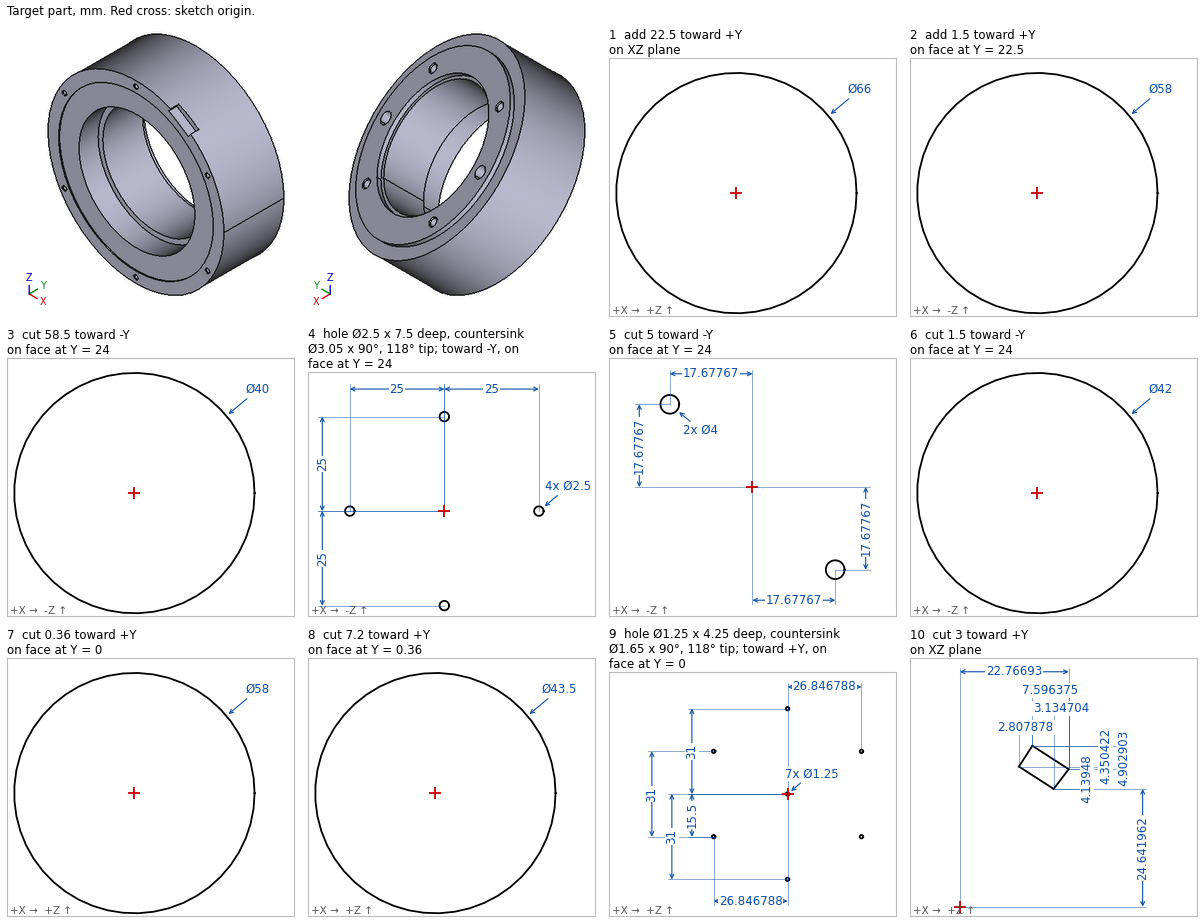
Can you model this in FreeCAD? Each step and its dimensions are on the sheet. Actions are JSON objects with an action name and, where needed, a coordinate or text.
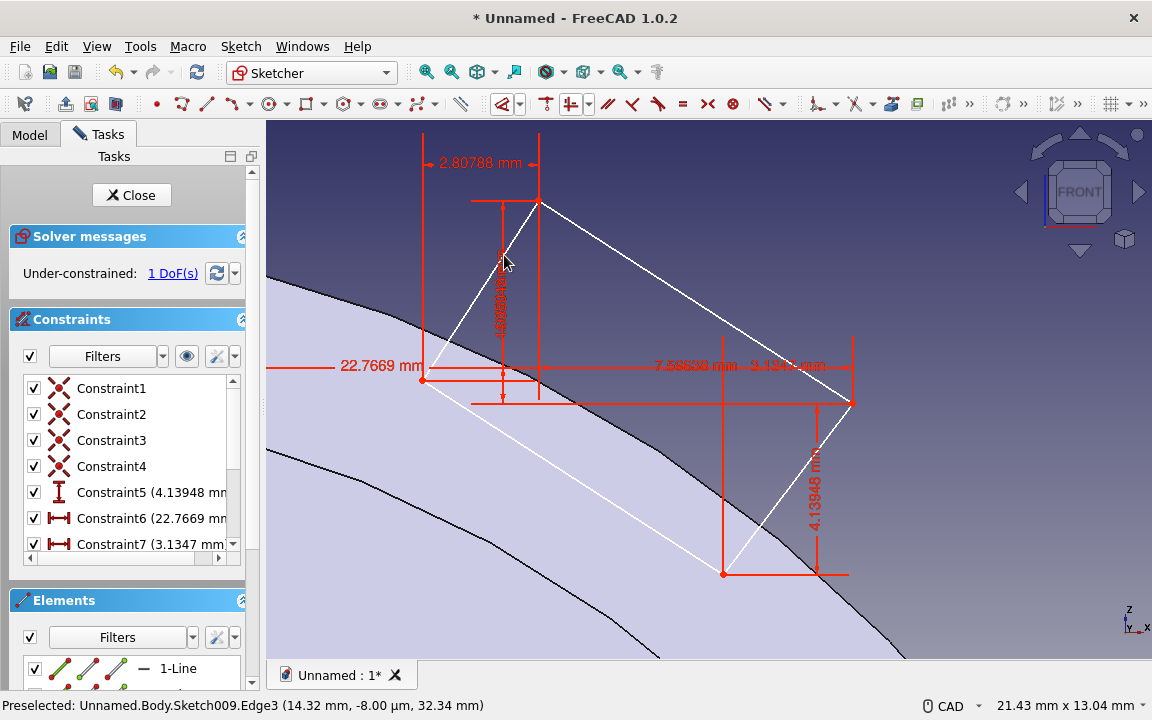
{"action": "left_click", "coordinate": [723, 575]}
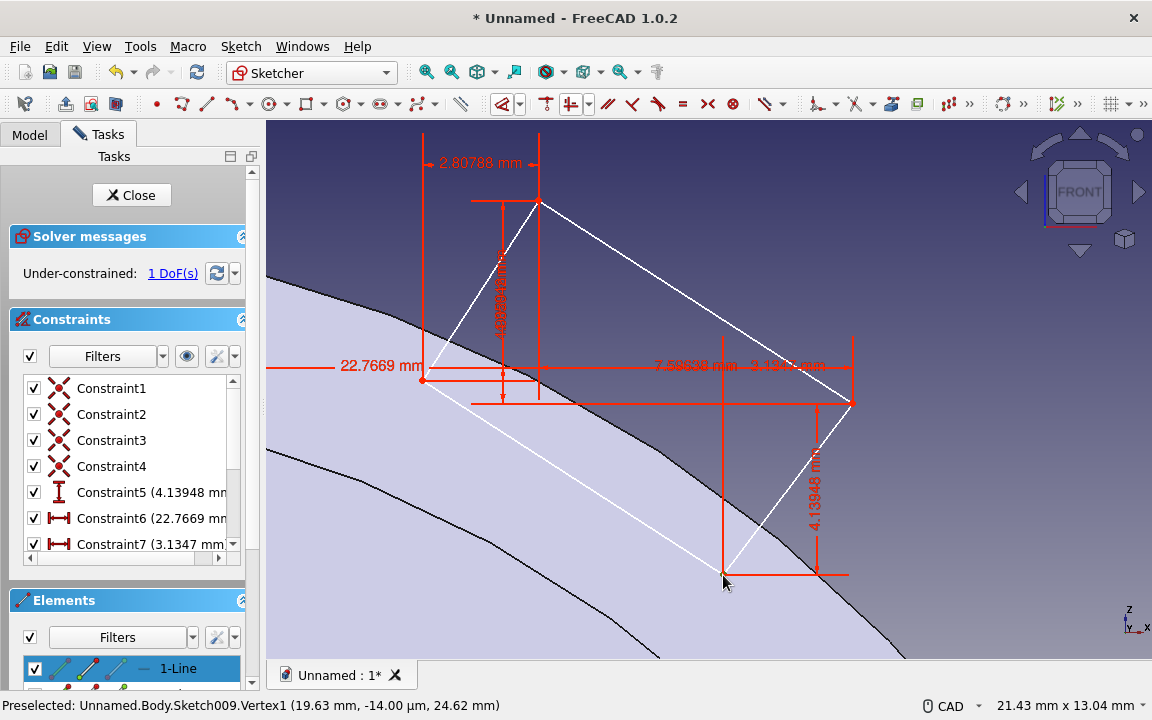
{"action": "key", "text": "i"}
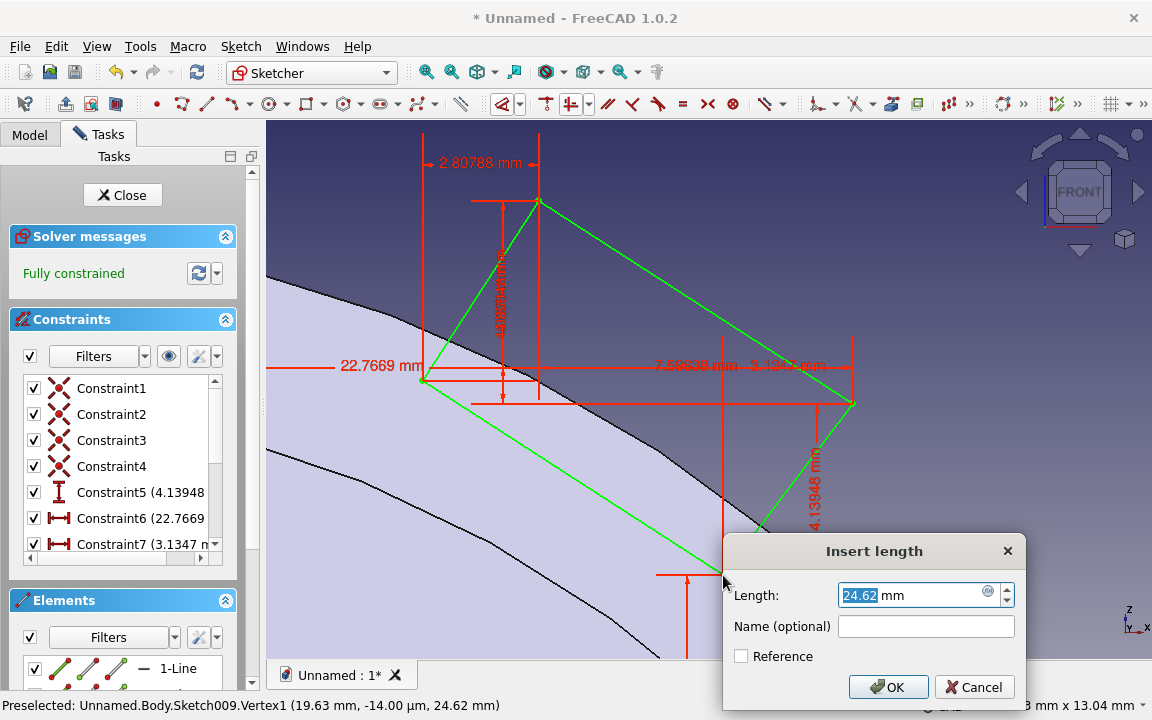
{"action": "type", "text": "24.641962"}
{"action": "key", "text": "Return"}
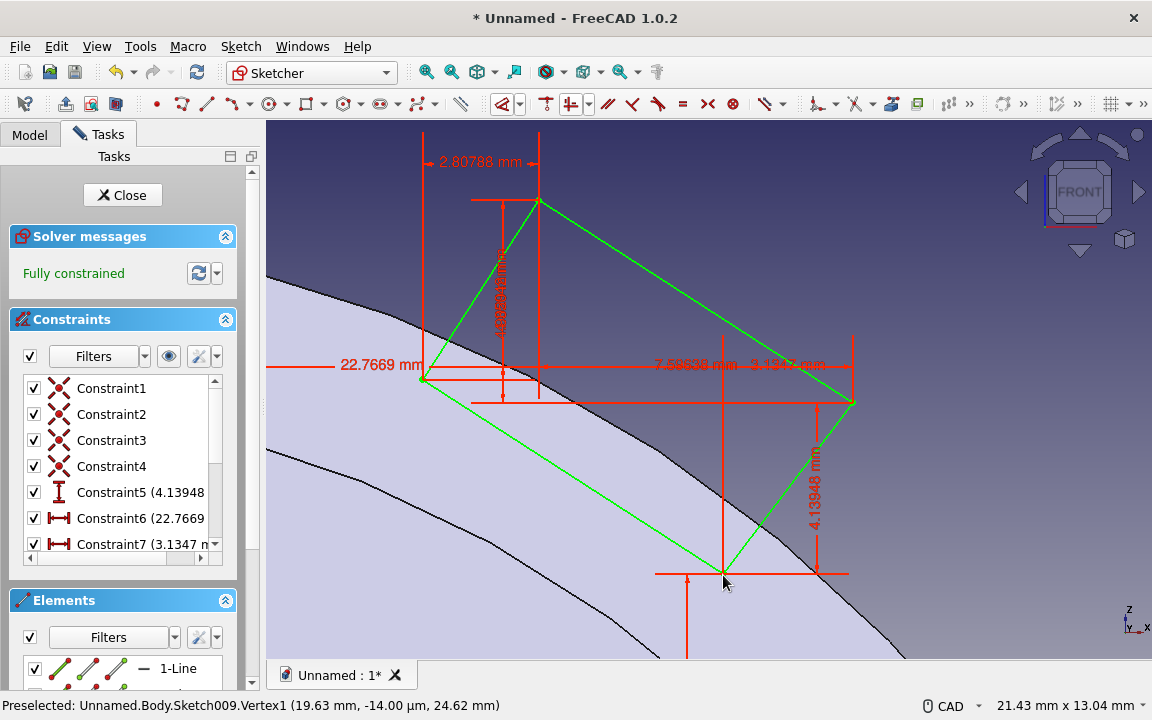
{"action": "left_click", "coordinate": [123, 195]}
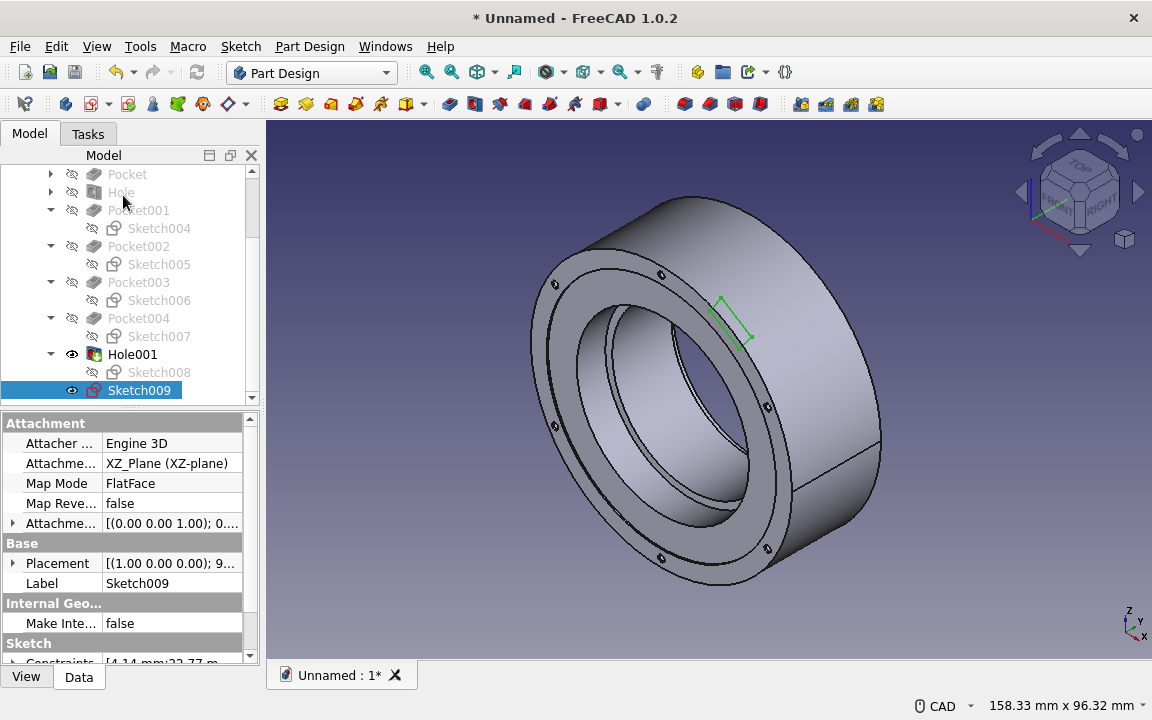
{"action": "left_click", "coordinate": [450, 104]}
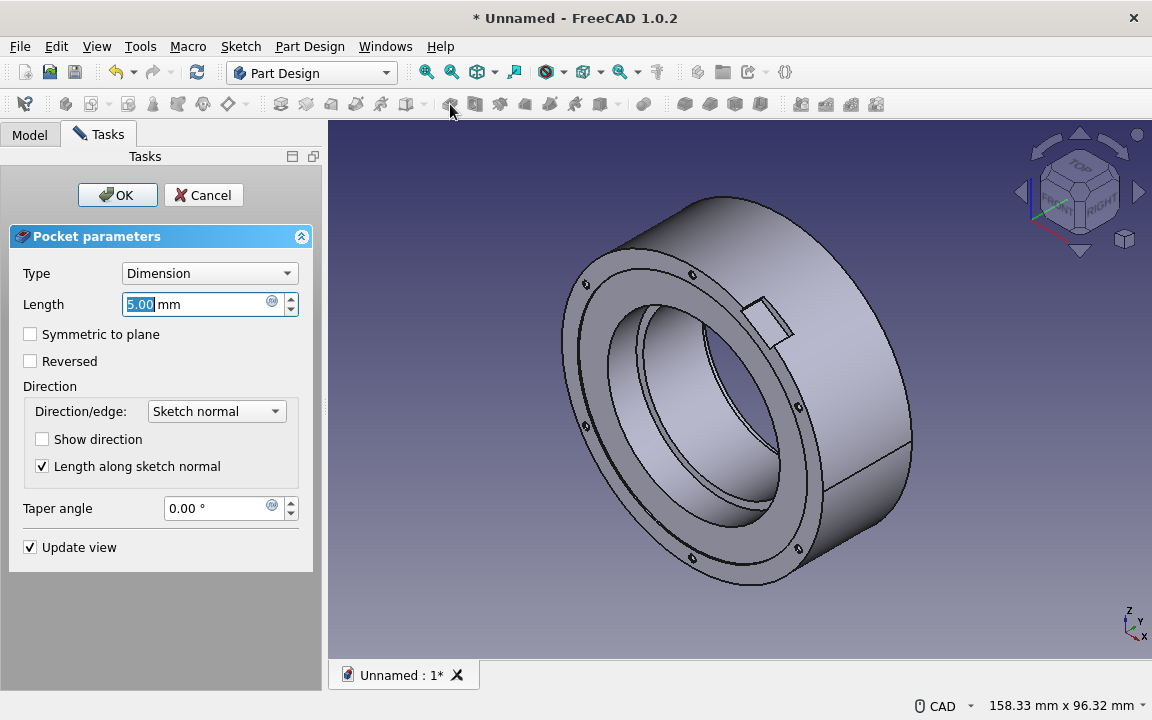
{"action": "type", "text": "3"}
{"action": "key", "text": "Tab"}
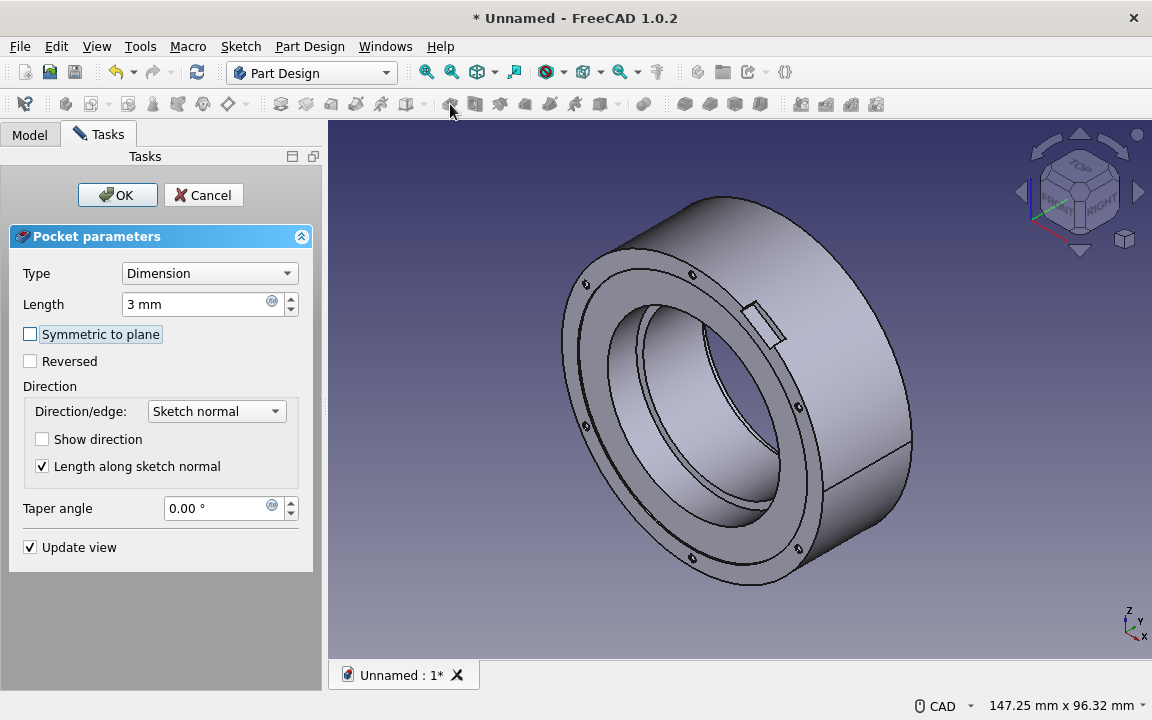
{"action": "left_click", "coordinate": [118, 195]}